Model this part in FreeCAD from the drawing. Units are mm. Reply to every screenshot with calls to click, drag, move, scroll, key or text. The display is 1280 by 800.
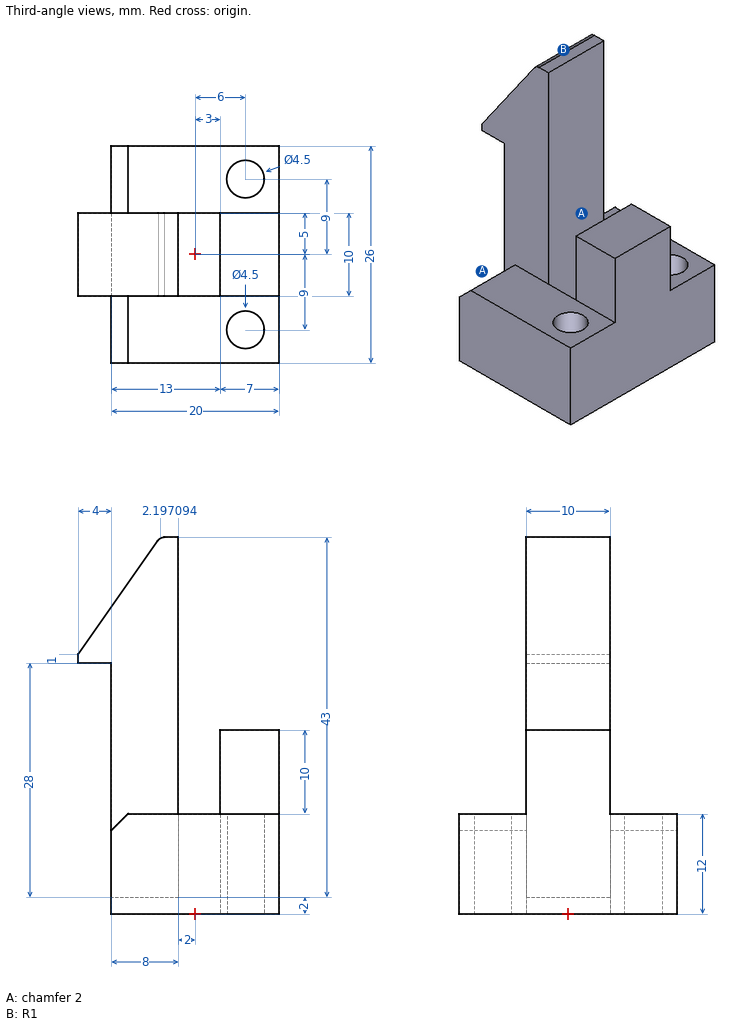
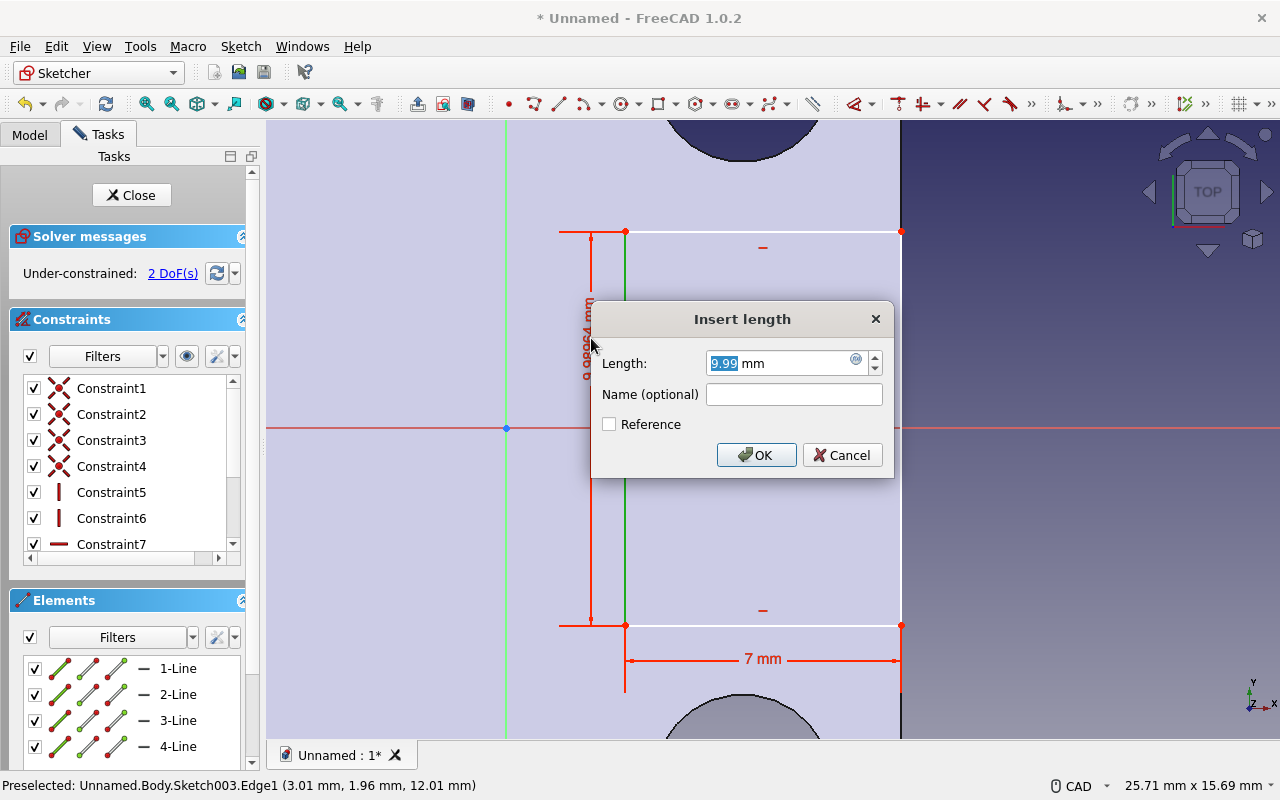
text(10)
key(Return)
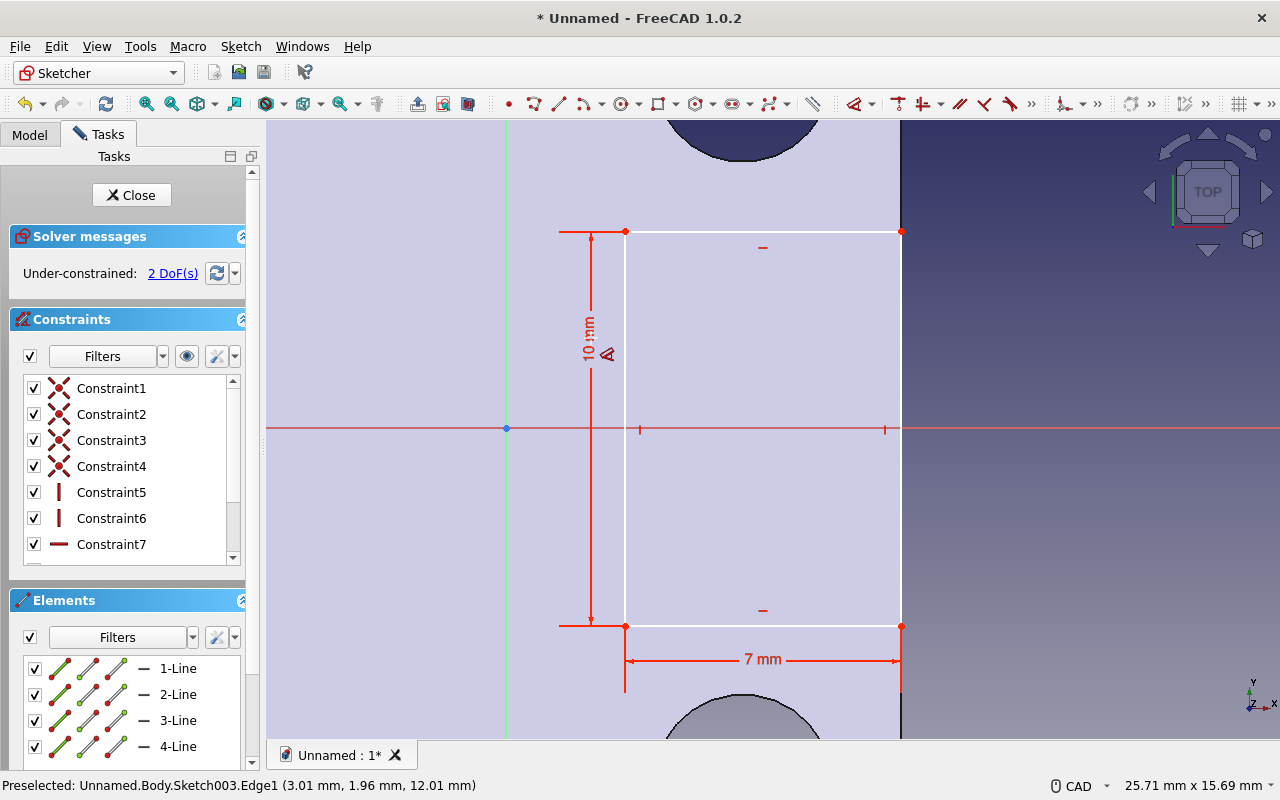
click(625, 232)
click(566, 198)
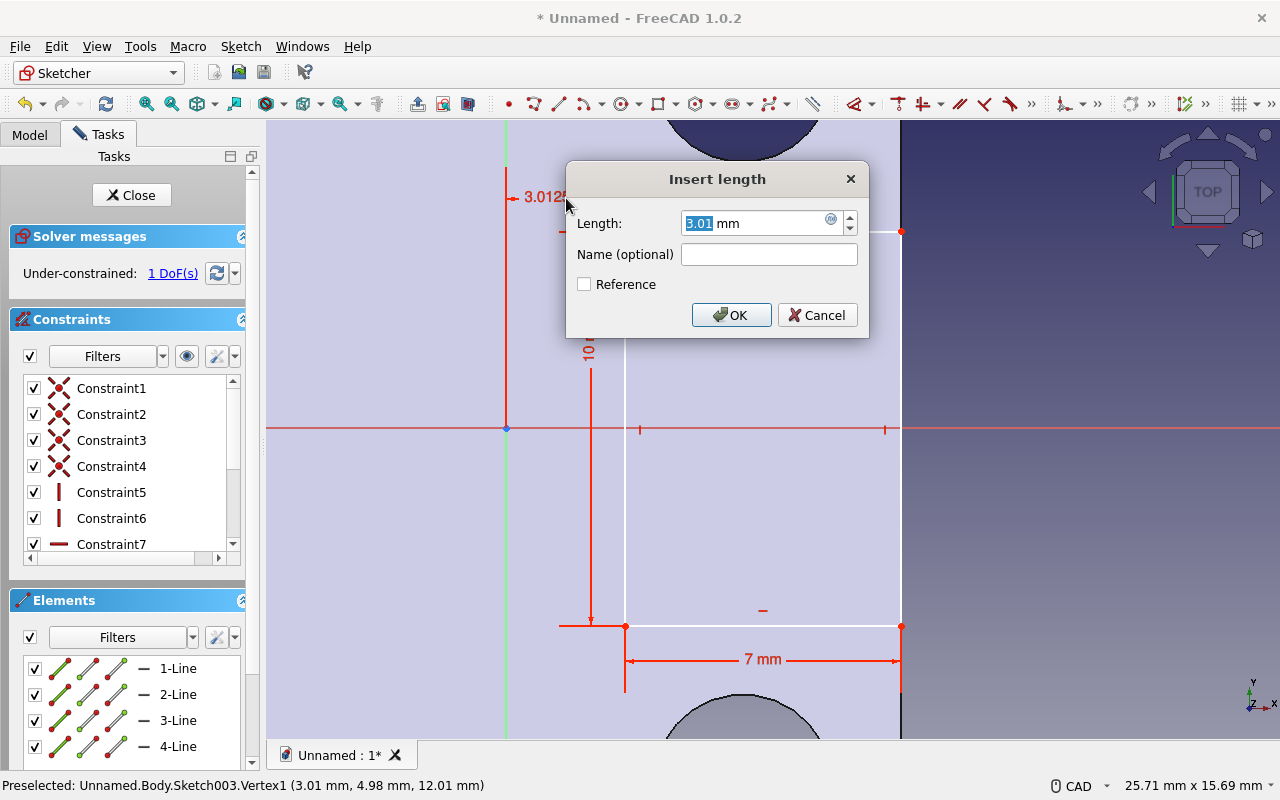
text(3)
key(Return)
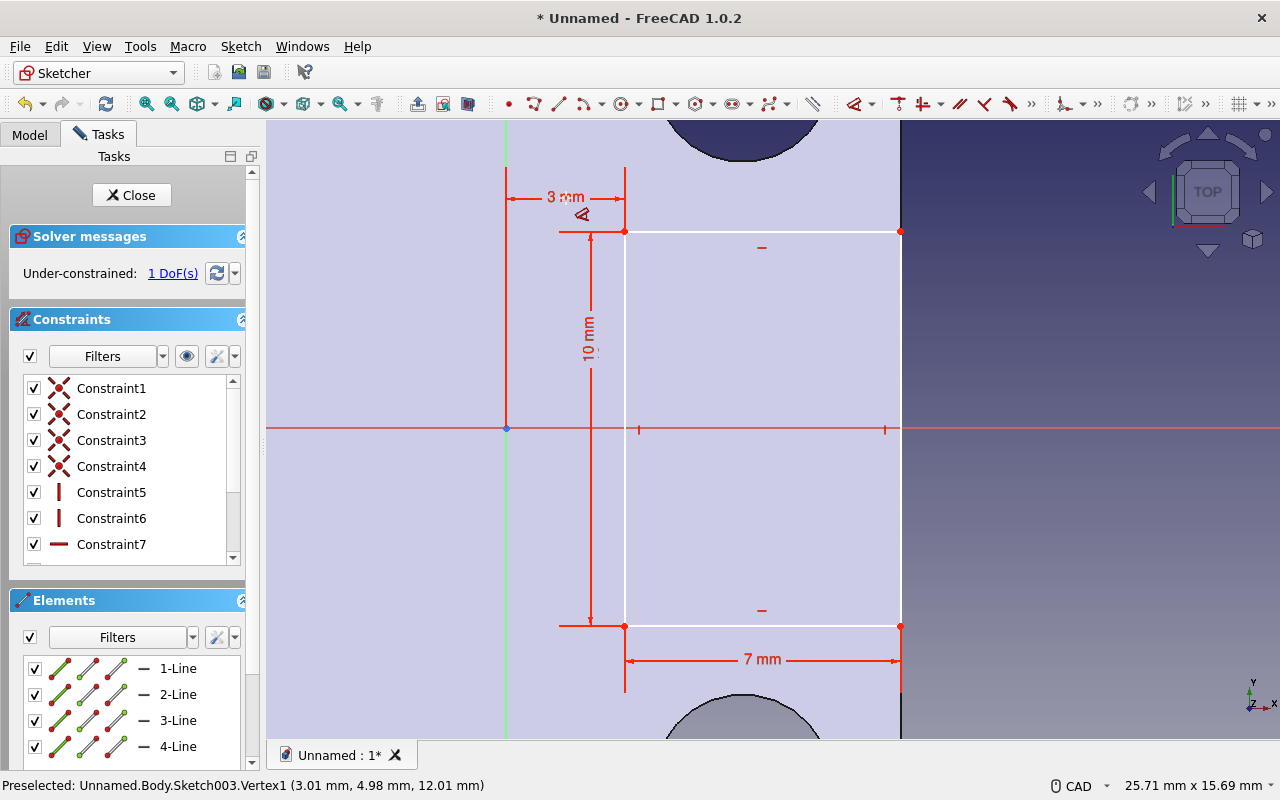
click(625, 232)
click(472, 330)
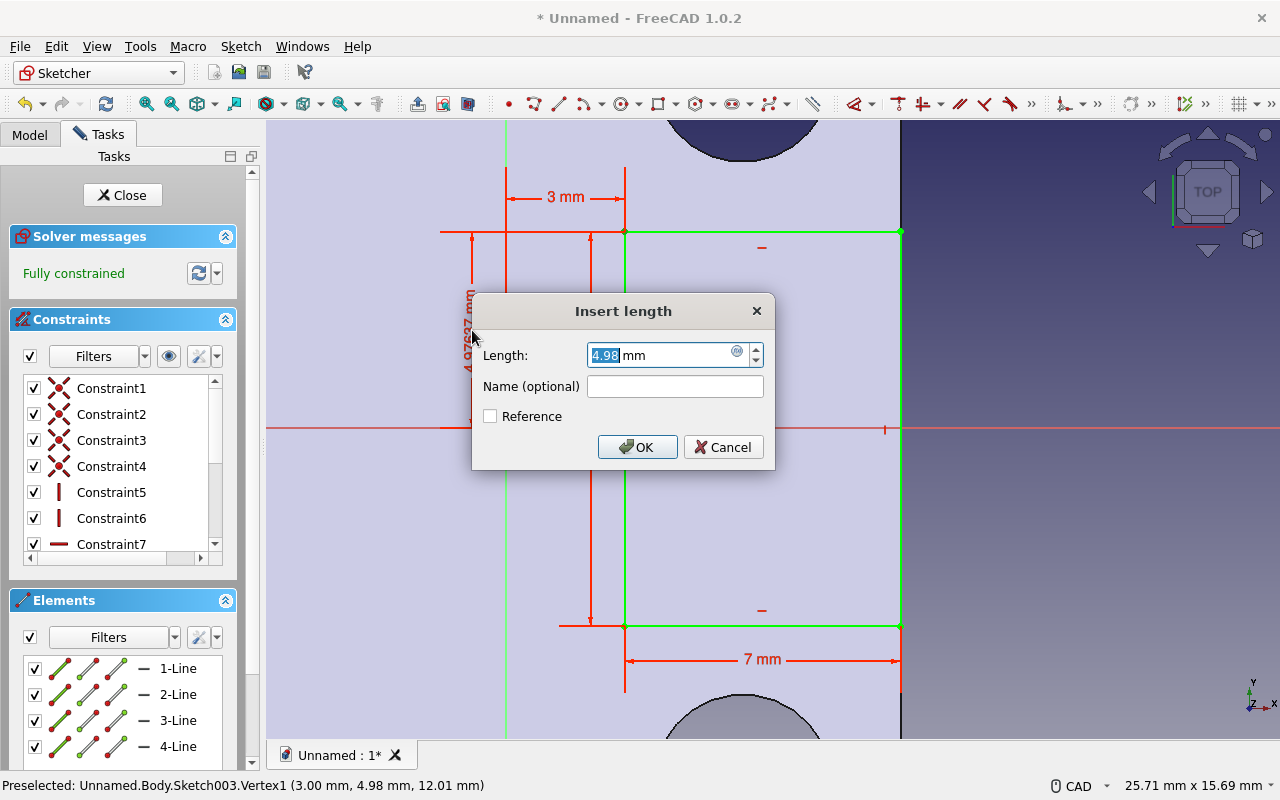
text(5)
key(Return)
key(Escape)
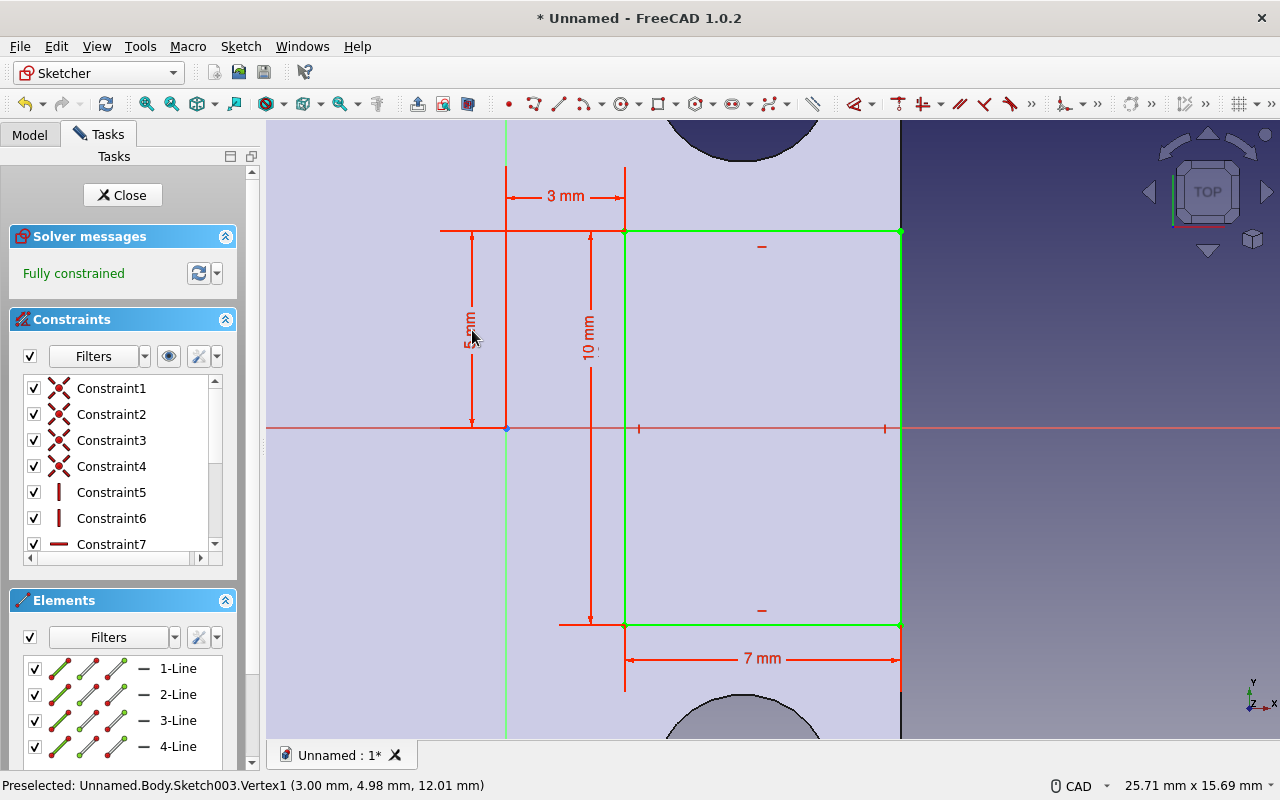
click(123, 195)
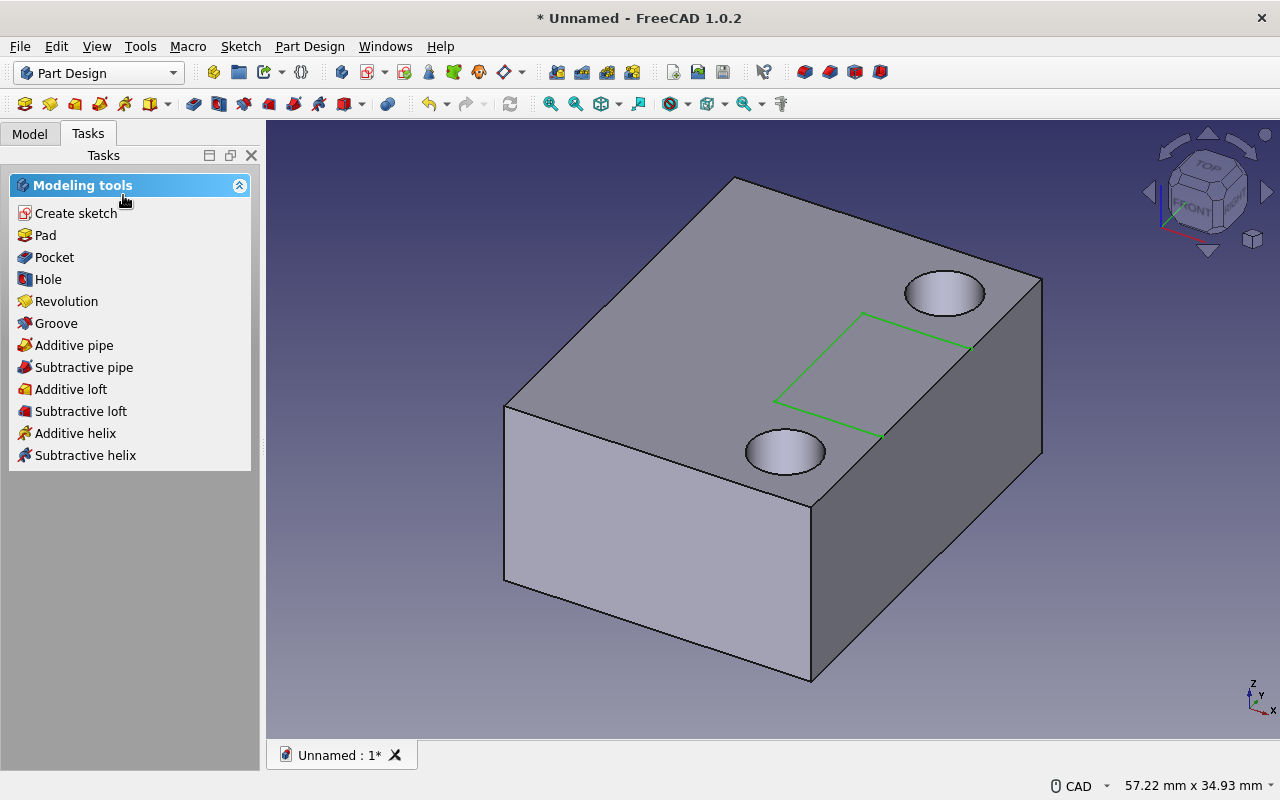
click(25, 104)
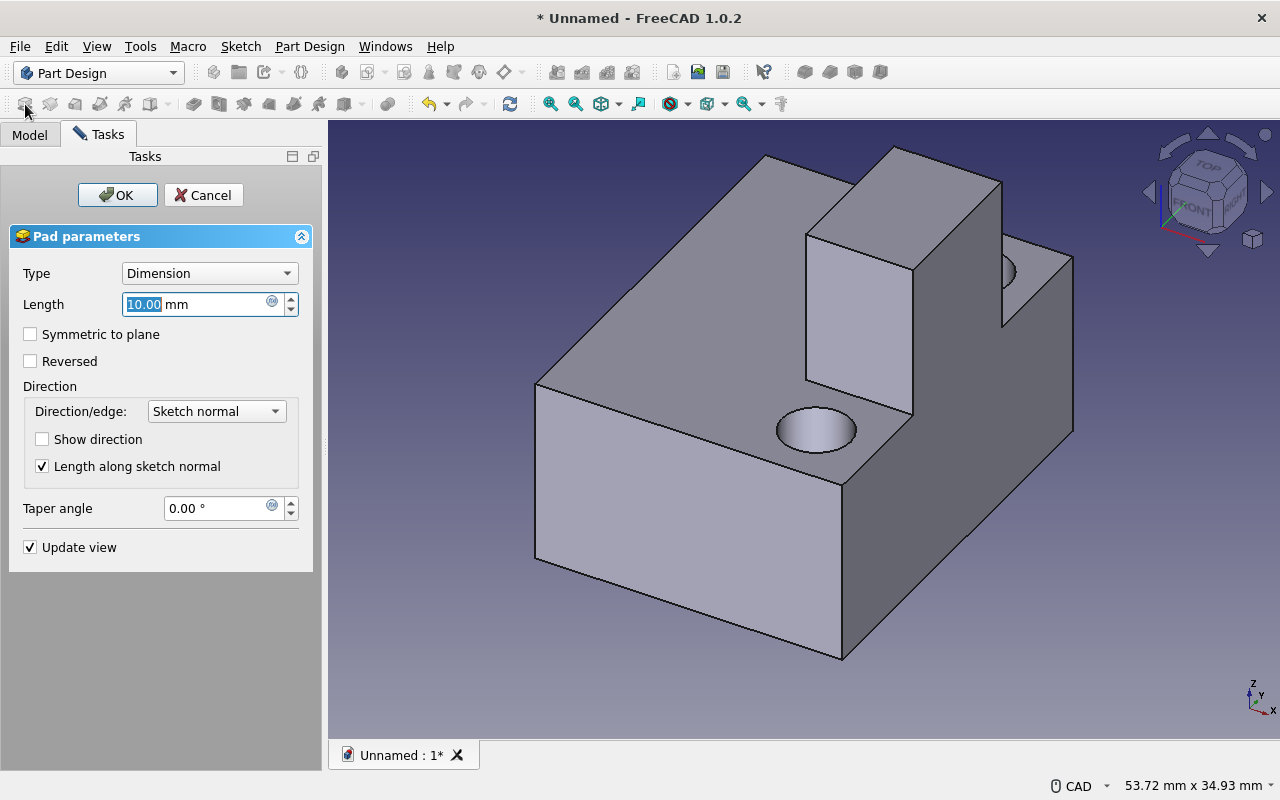
text(10)
key(Tab)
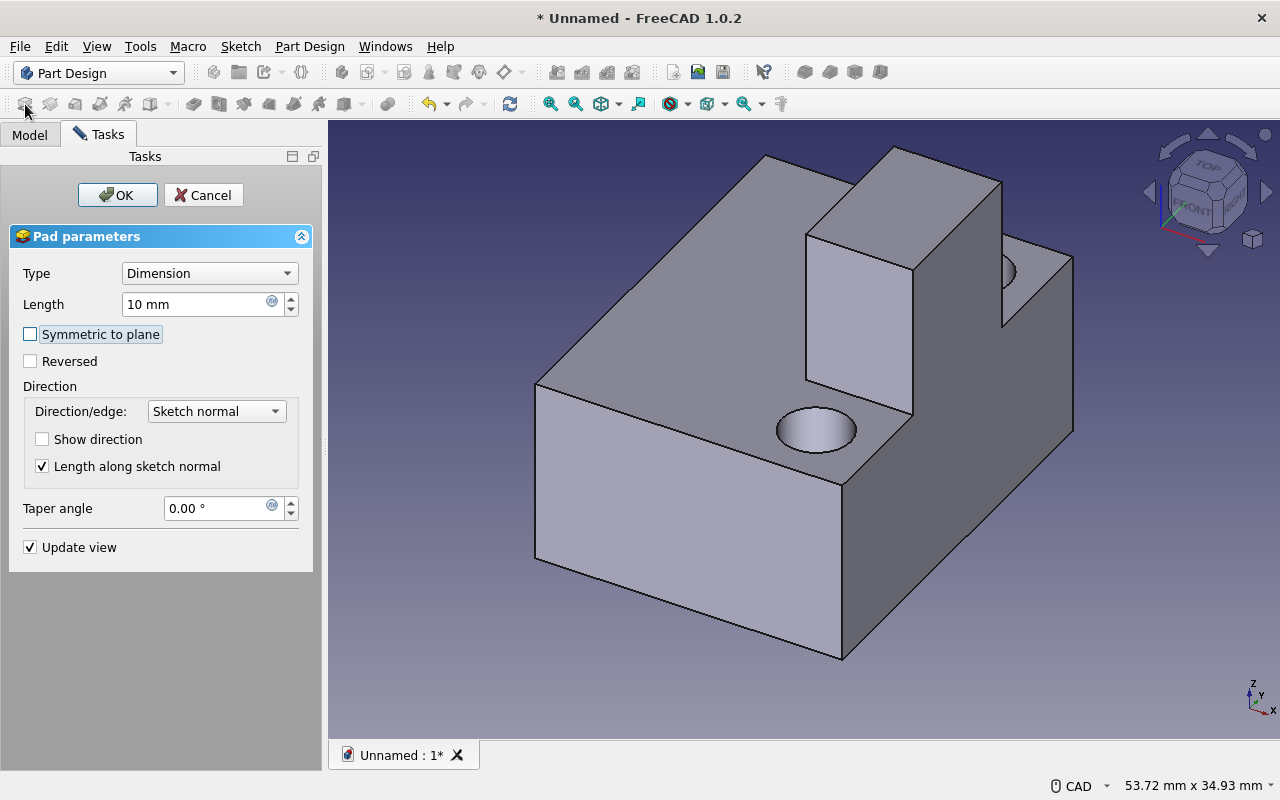
click(118, 195)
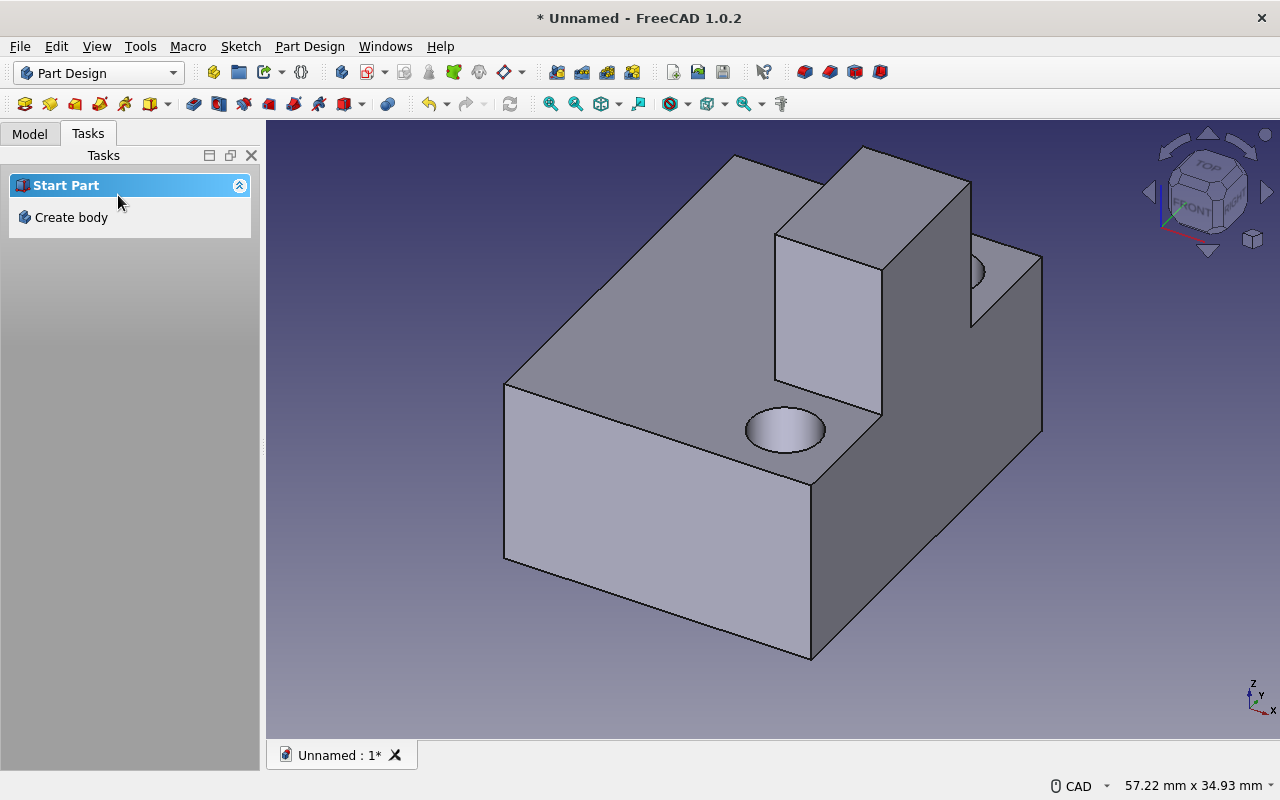
click(551, 104)